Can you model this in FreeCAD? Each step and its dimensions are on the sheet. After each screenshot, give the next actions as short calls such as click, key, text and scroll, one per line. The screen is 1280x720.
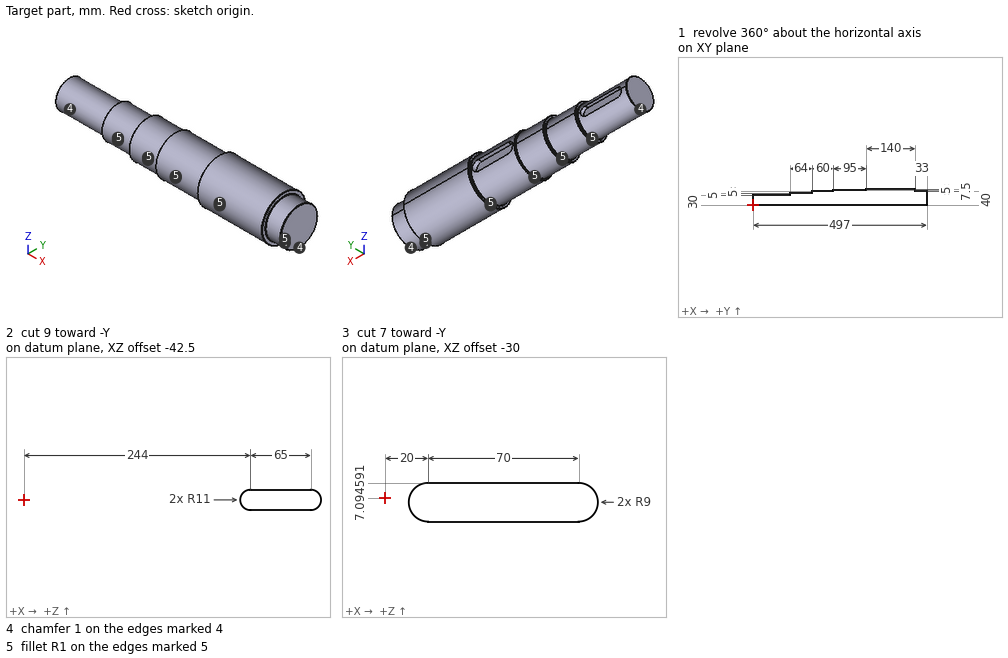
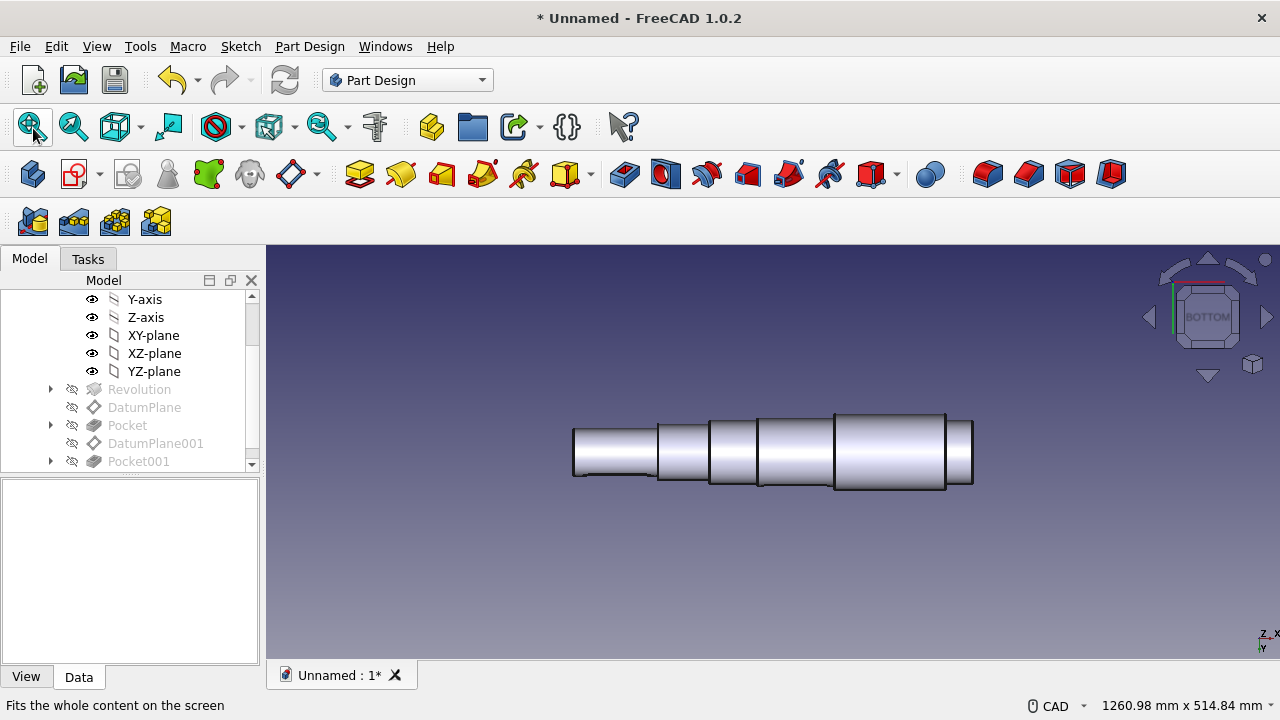
click(33, 128)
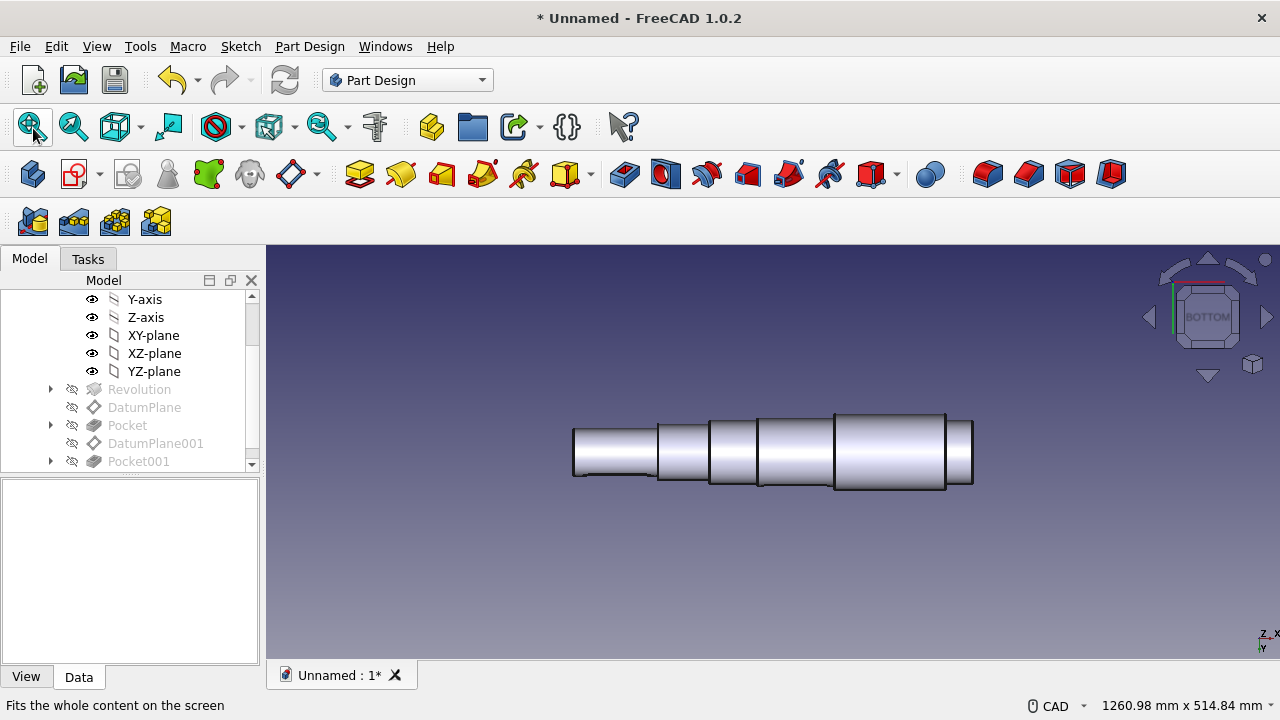
key(4)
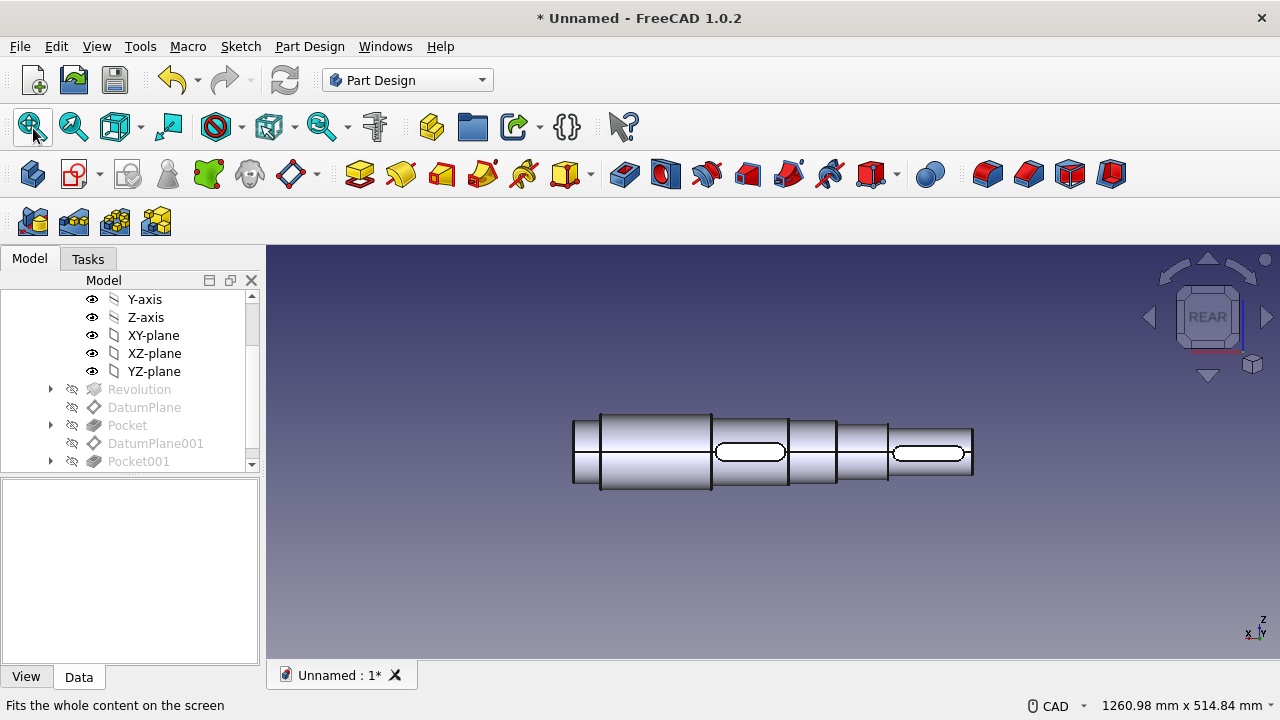
click(33, 128)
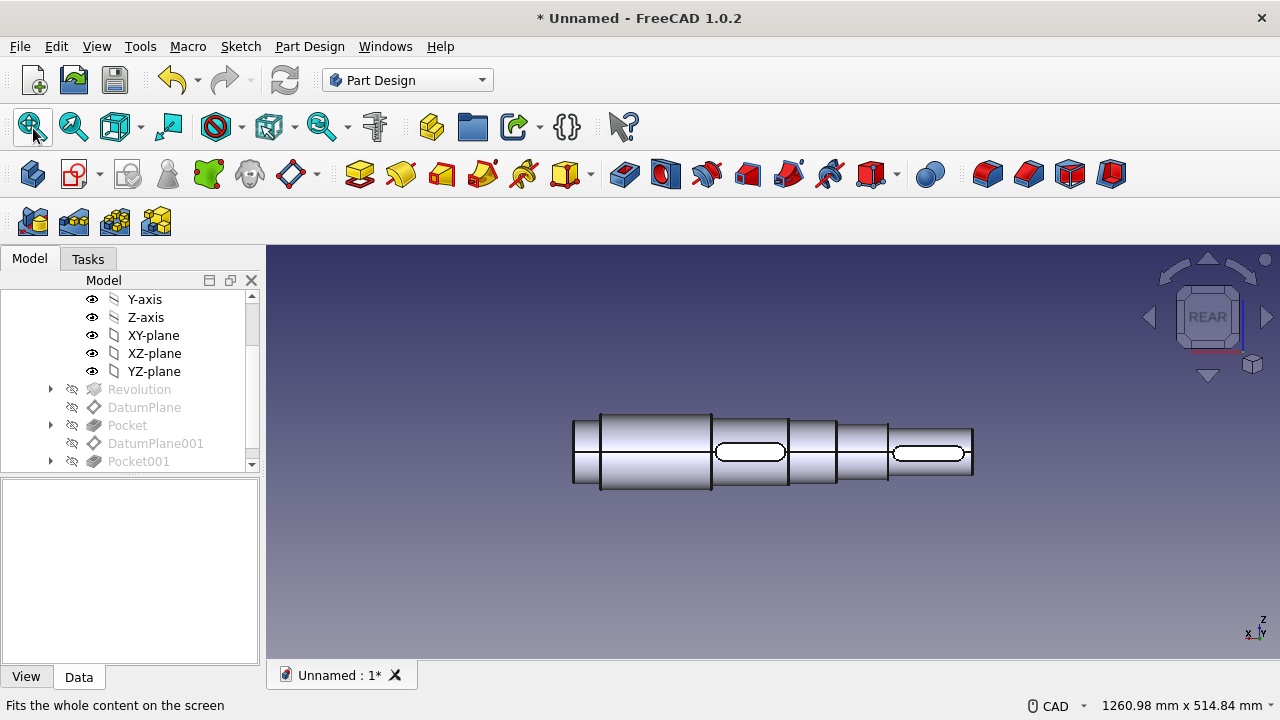
key(6)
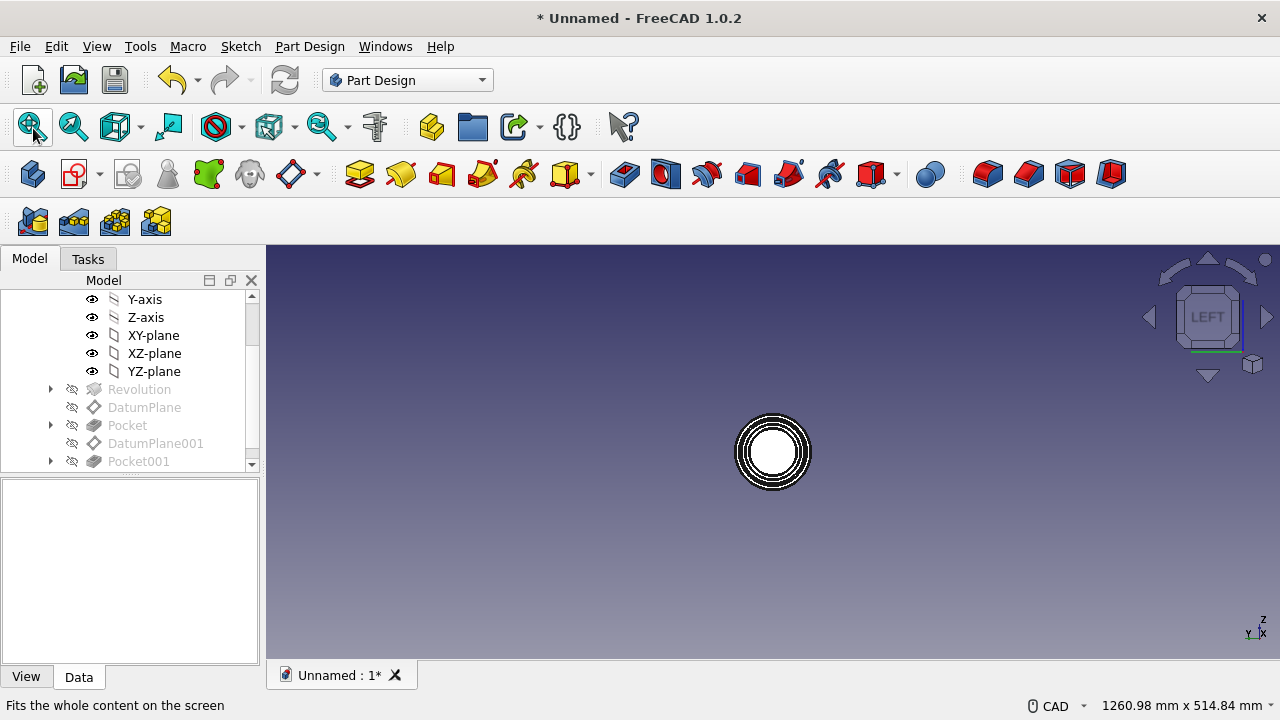
click(33, 128)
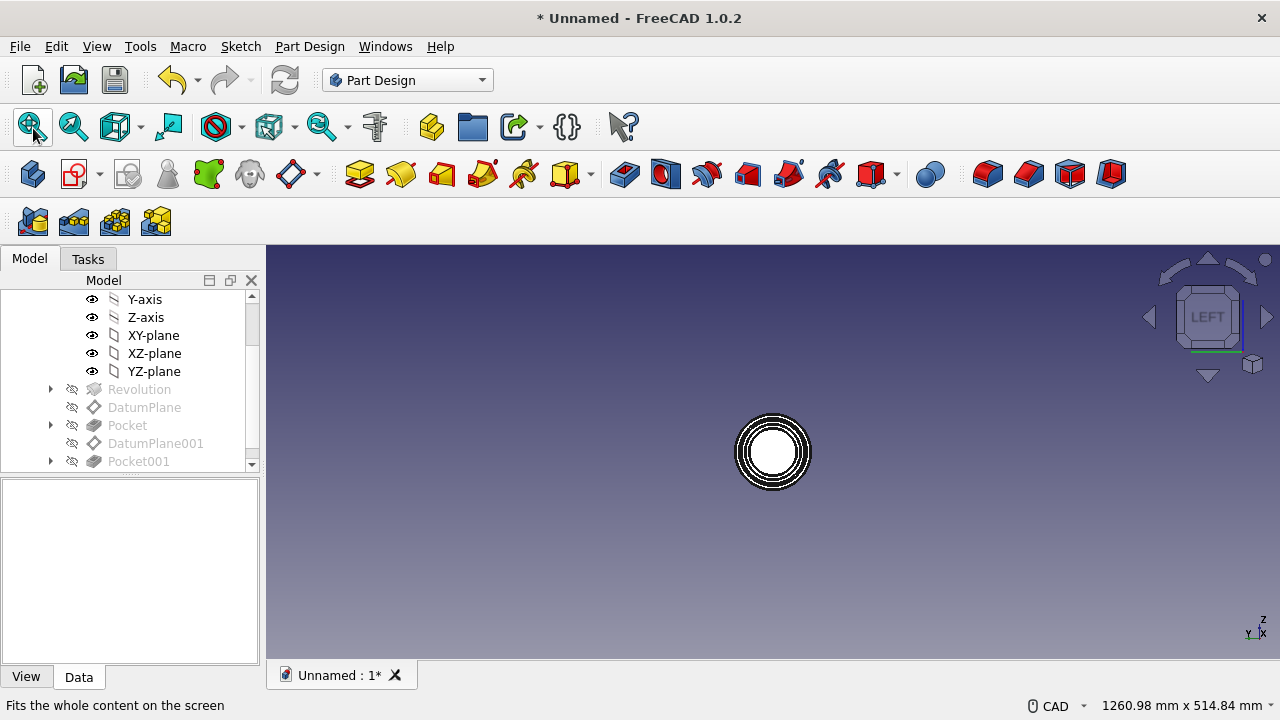
key(v)
key(3)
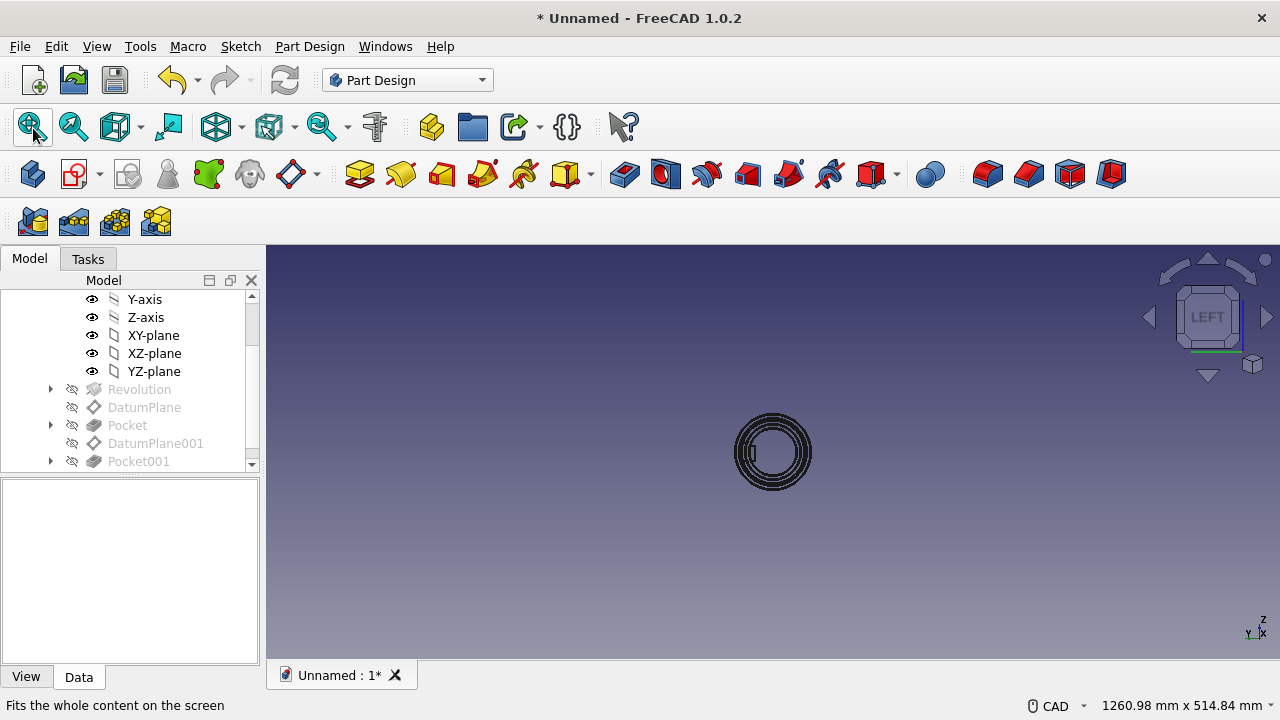
key(0)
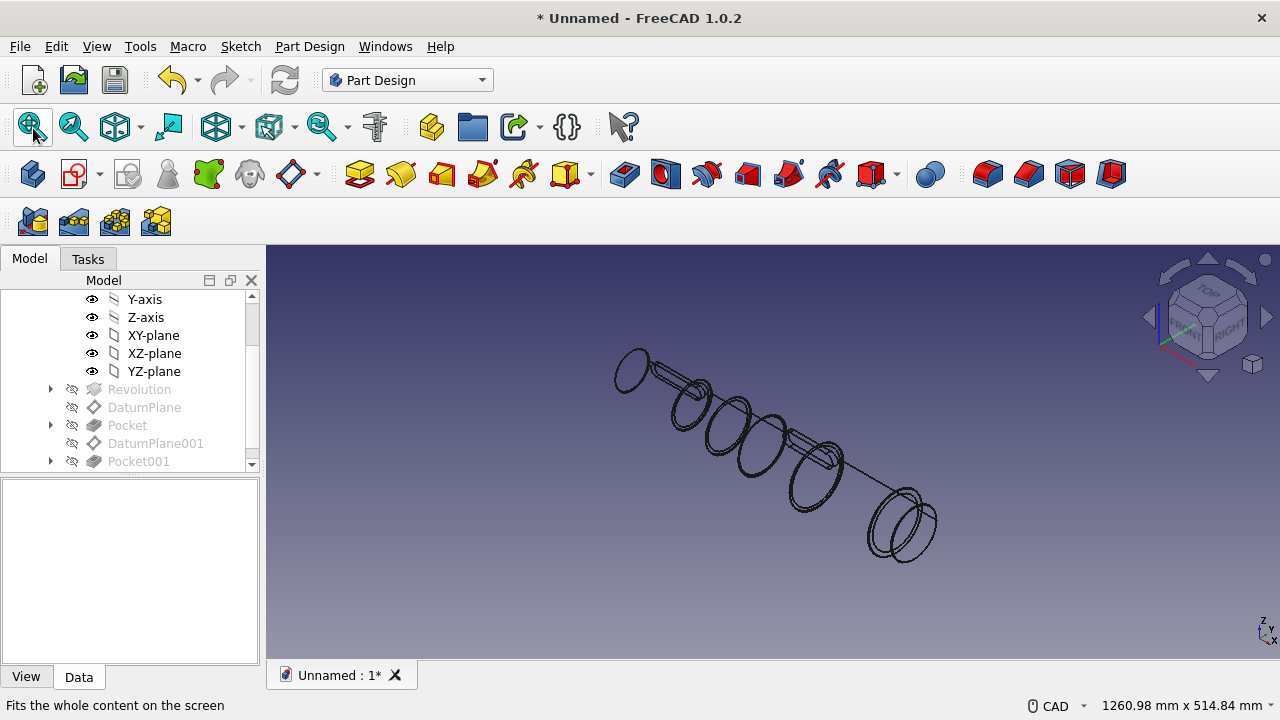
click(903, 543)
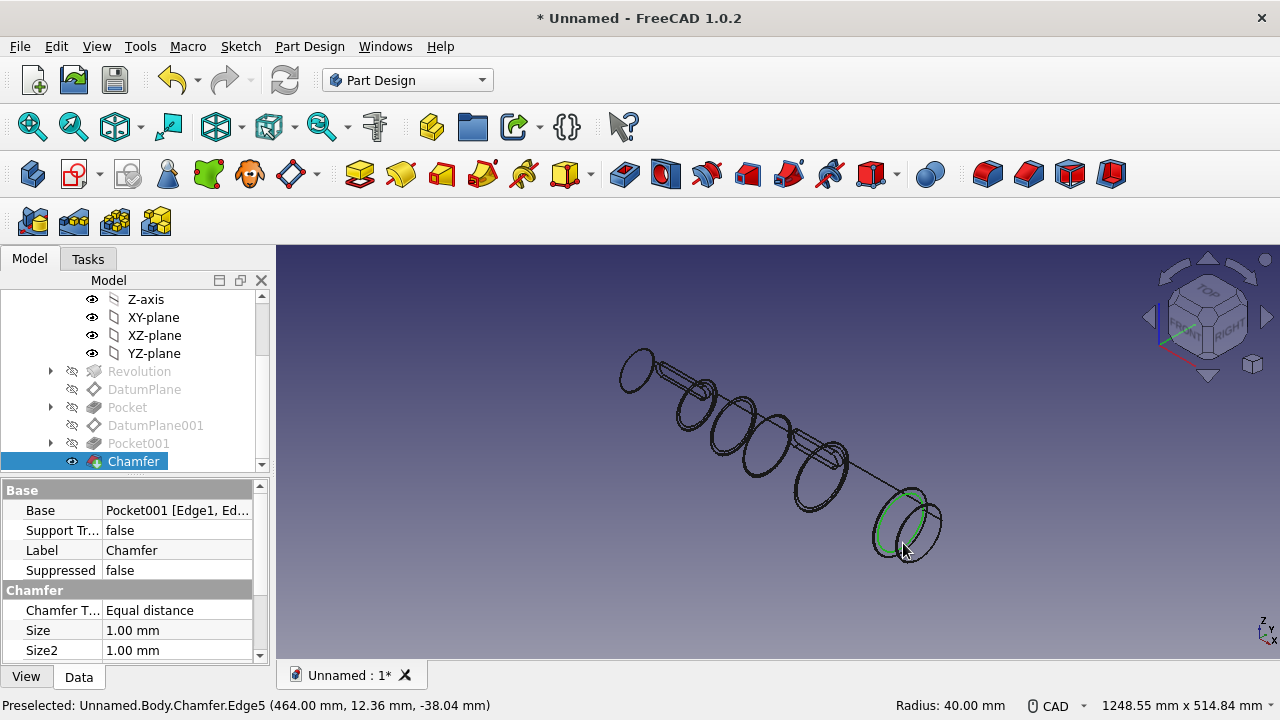
click(813, 507, ctrl)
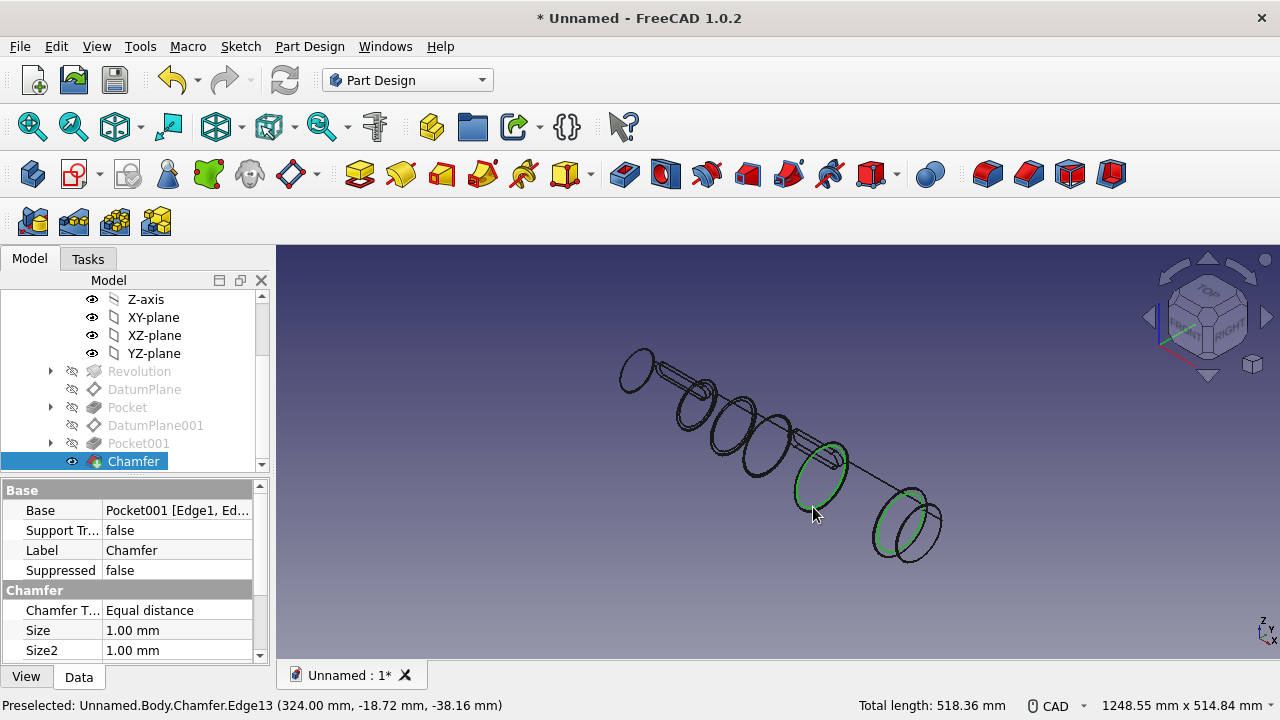
click(783, 453, ctrl)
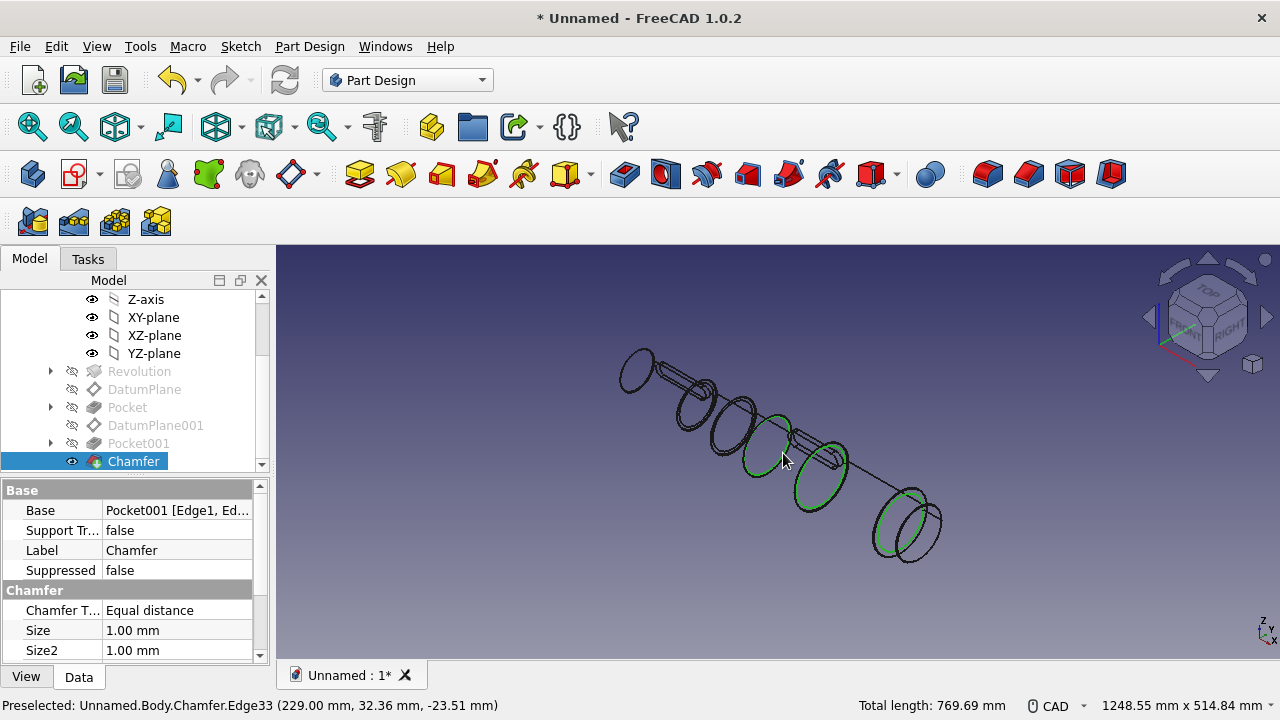
click(739, 443, ctrl)